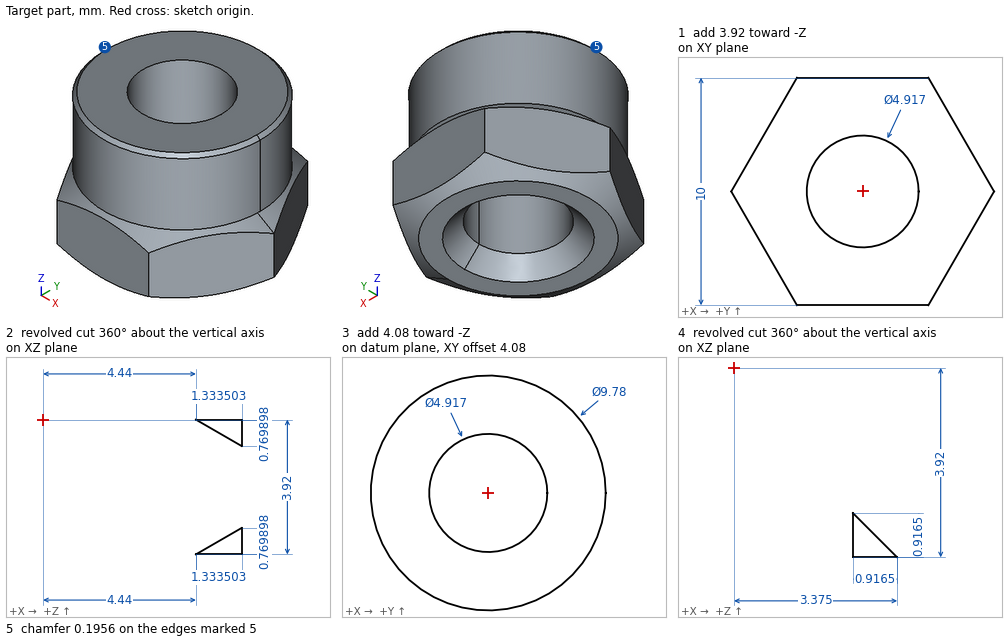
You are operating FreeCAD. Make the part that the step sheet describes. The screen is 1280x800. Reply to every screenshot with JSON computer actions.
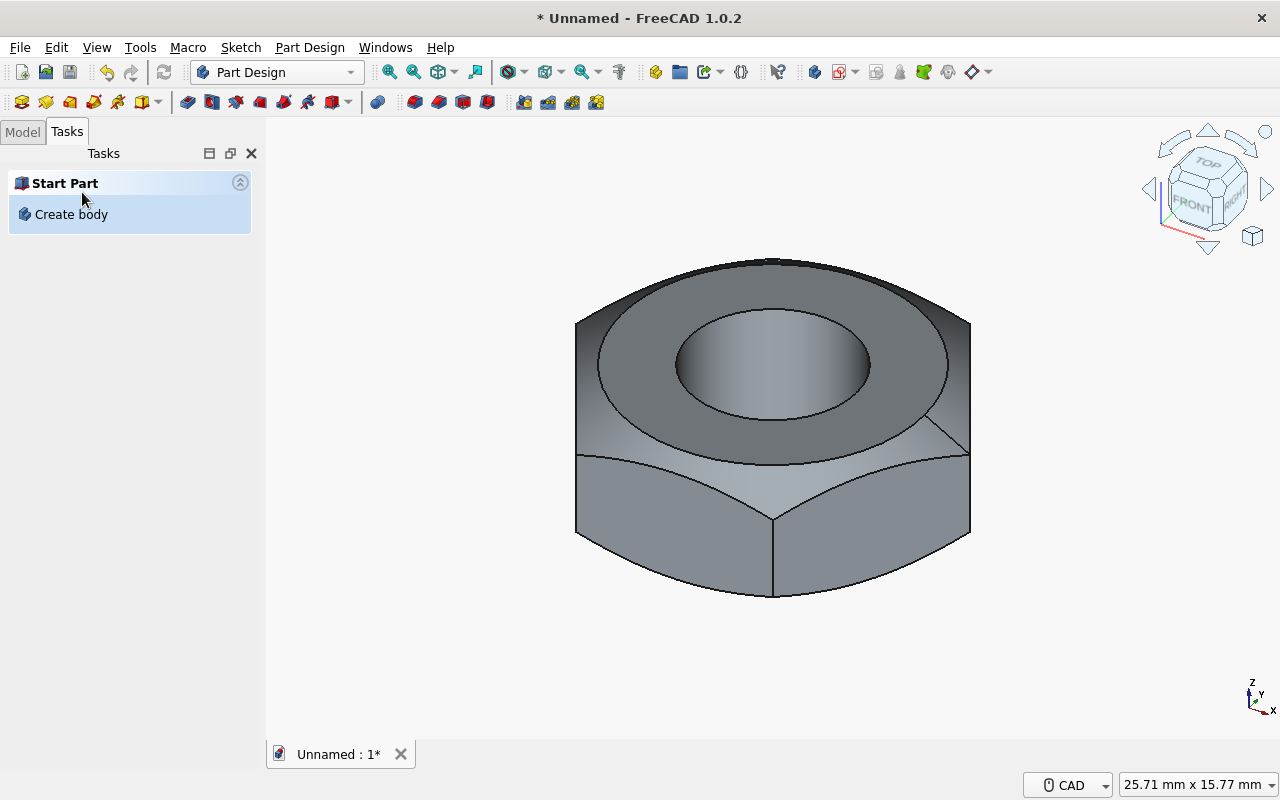
{"action": "left_click", "coordinate": [23, 131]}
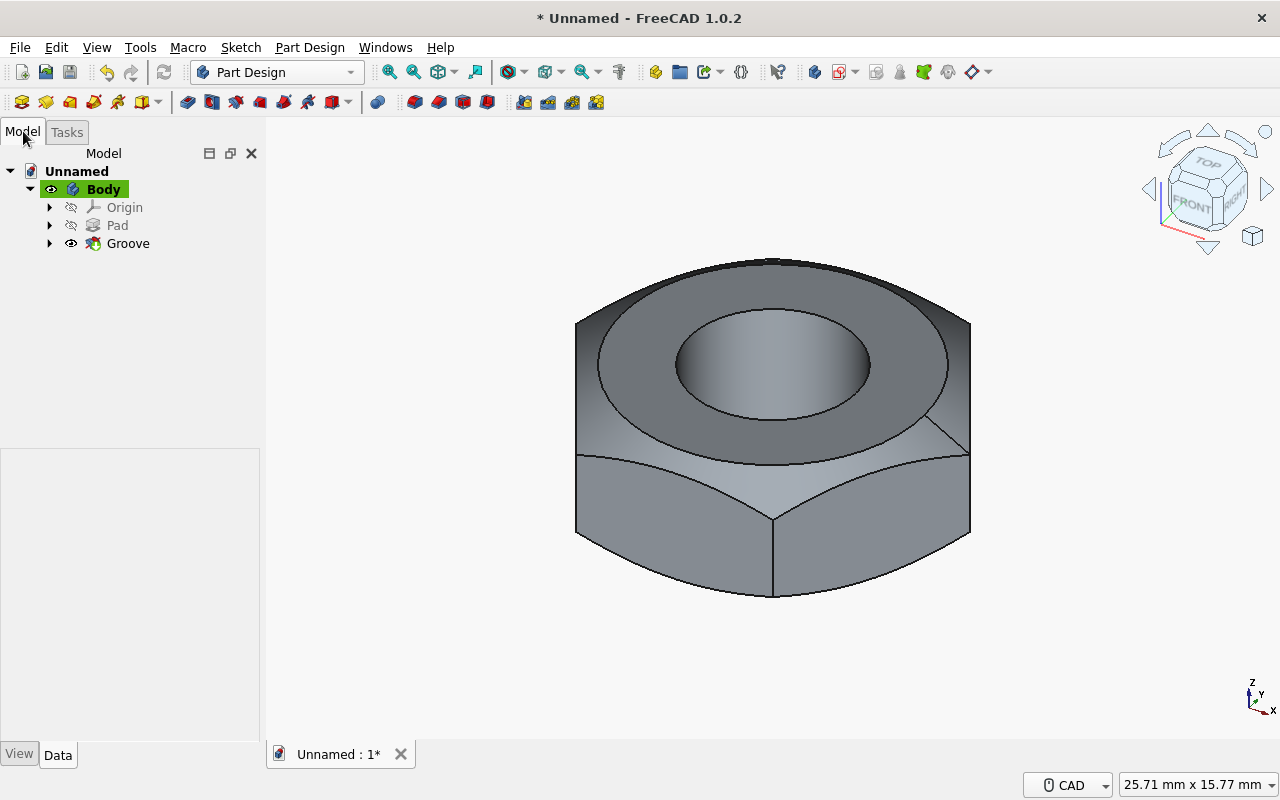
{"action": "left_click", "coordinate": [50, 207]}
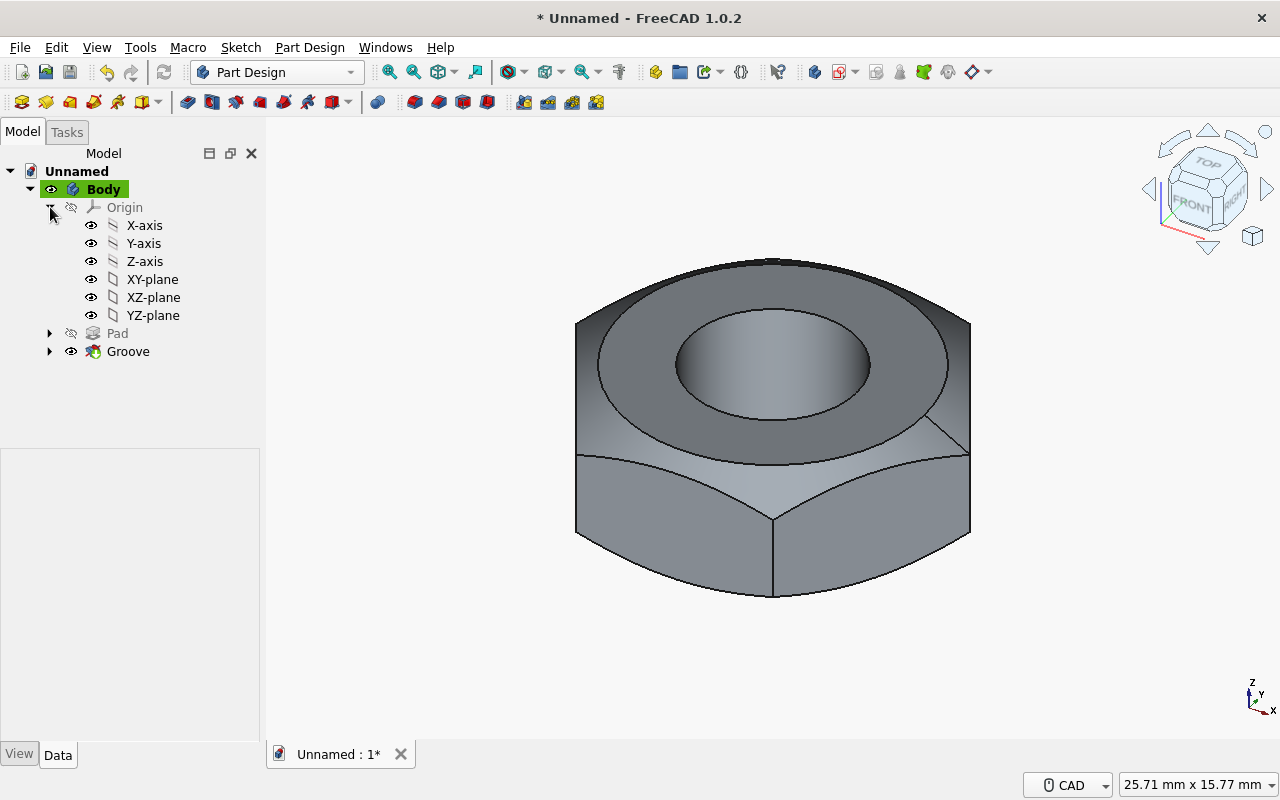
{"action": "left_click", "coordinate": [136, 279]}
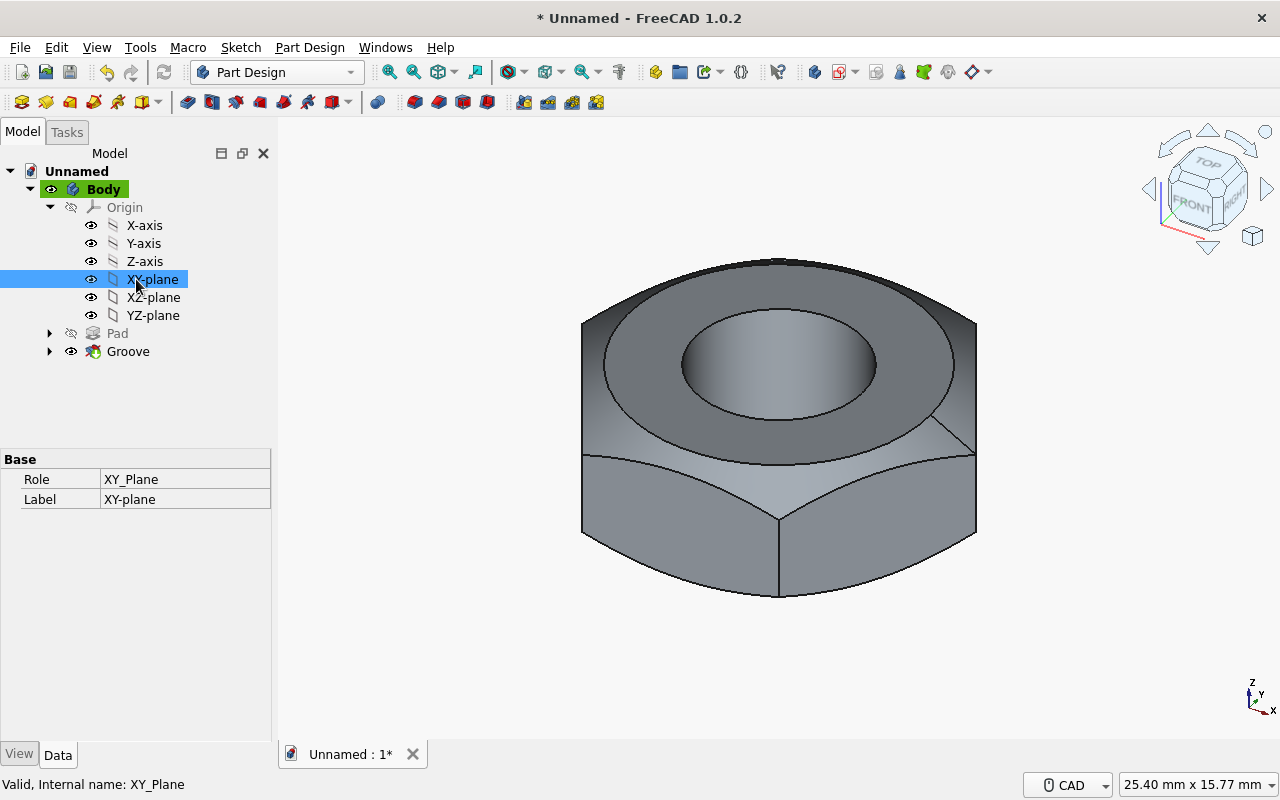
{"action": "left_click", "coordinate": [972, 72]}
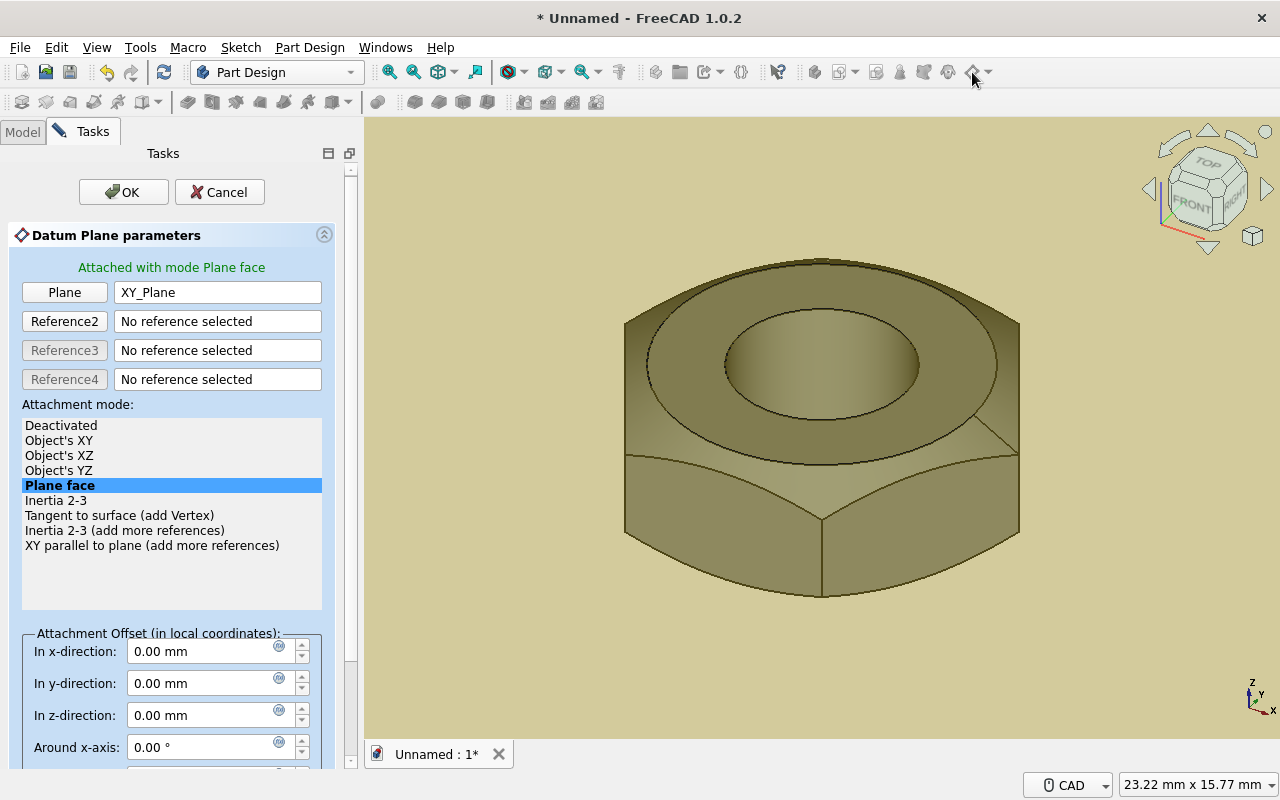
{"action": "triple_click", "coordinate": [210, 715]}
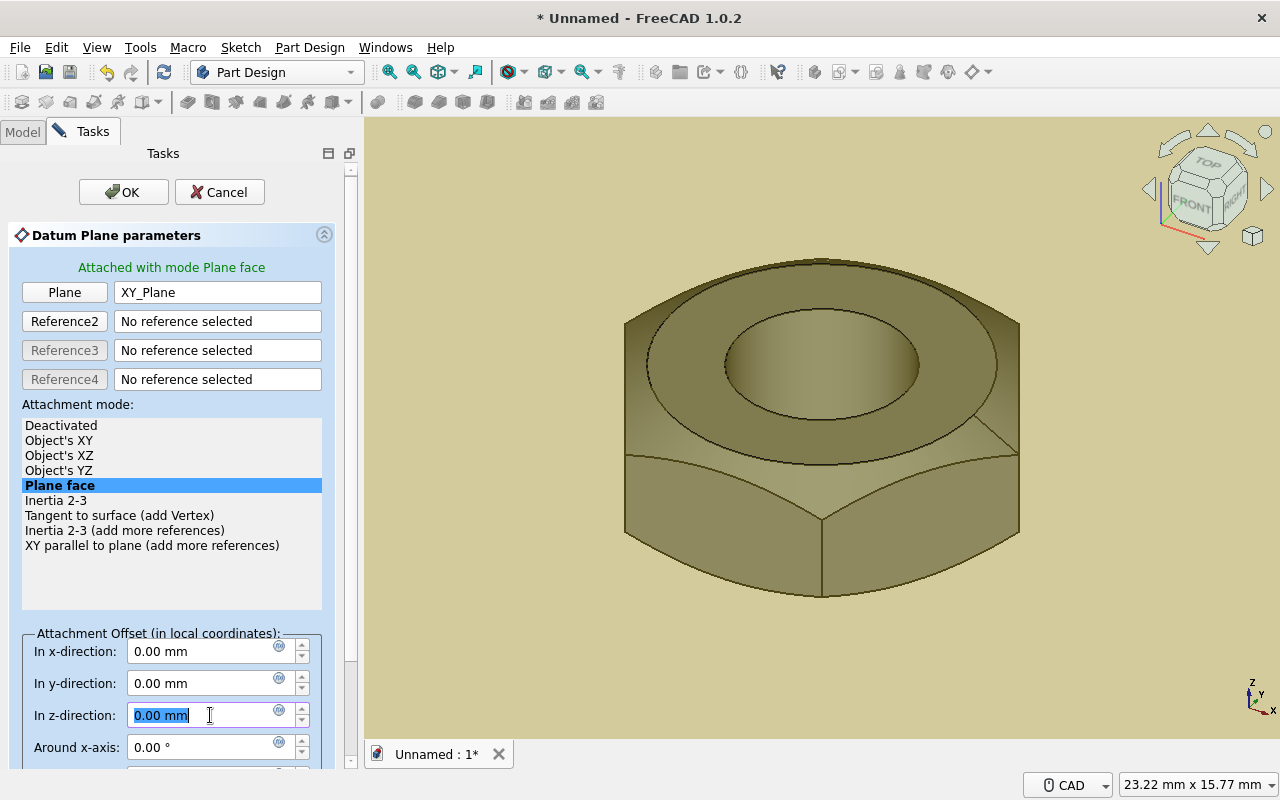
{"action": "type", "text": "4.08"}
{"action": "key", "text": "Tab"}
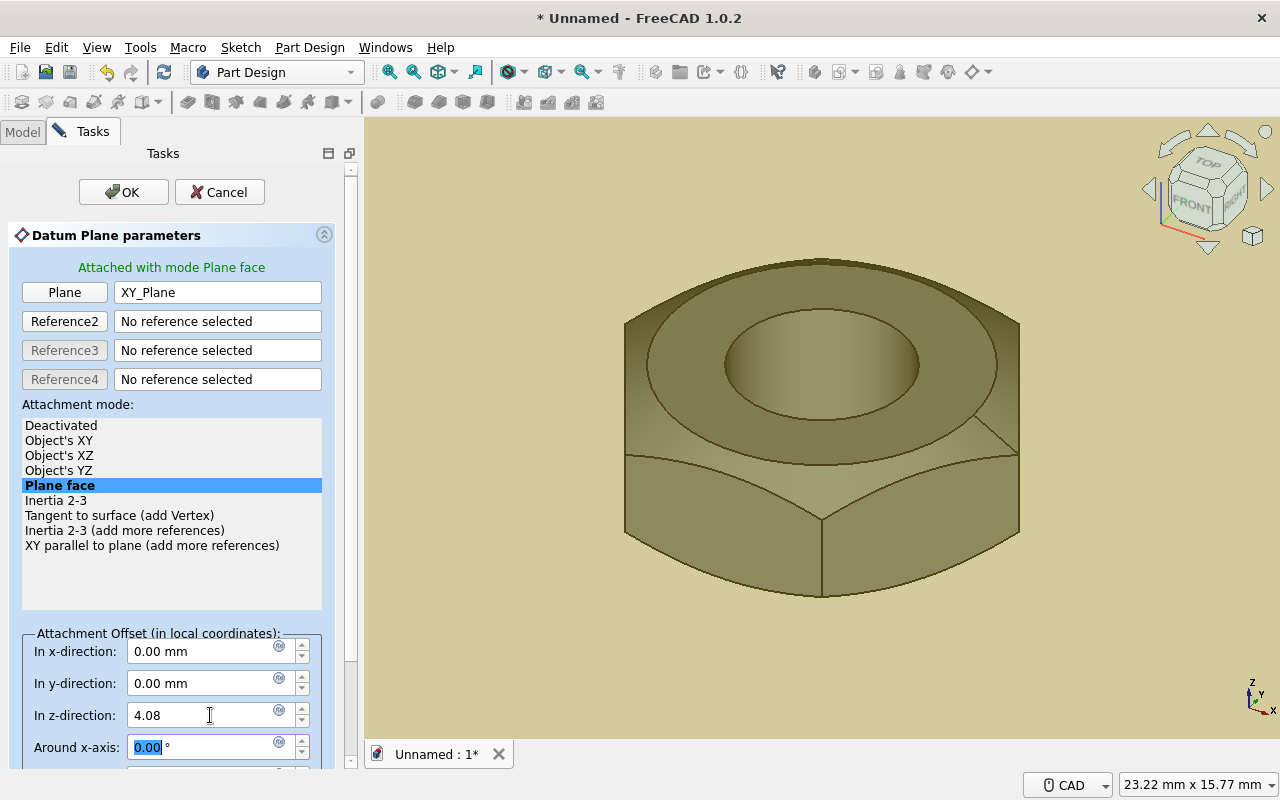
{"action": "left_click", "coordinate": [124, 192]}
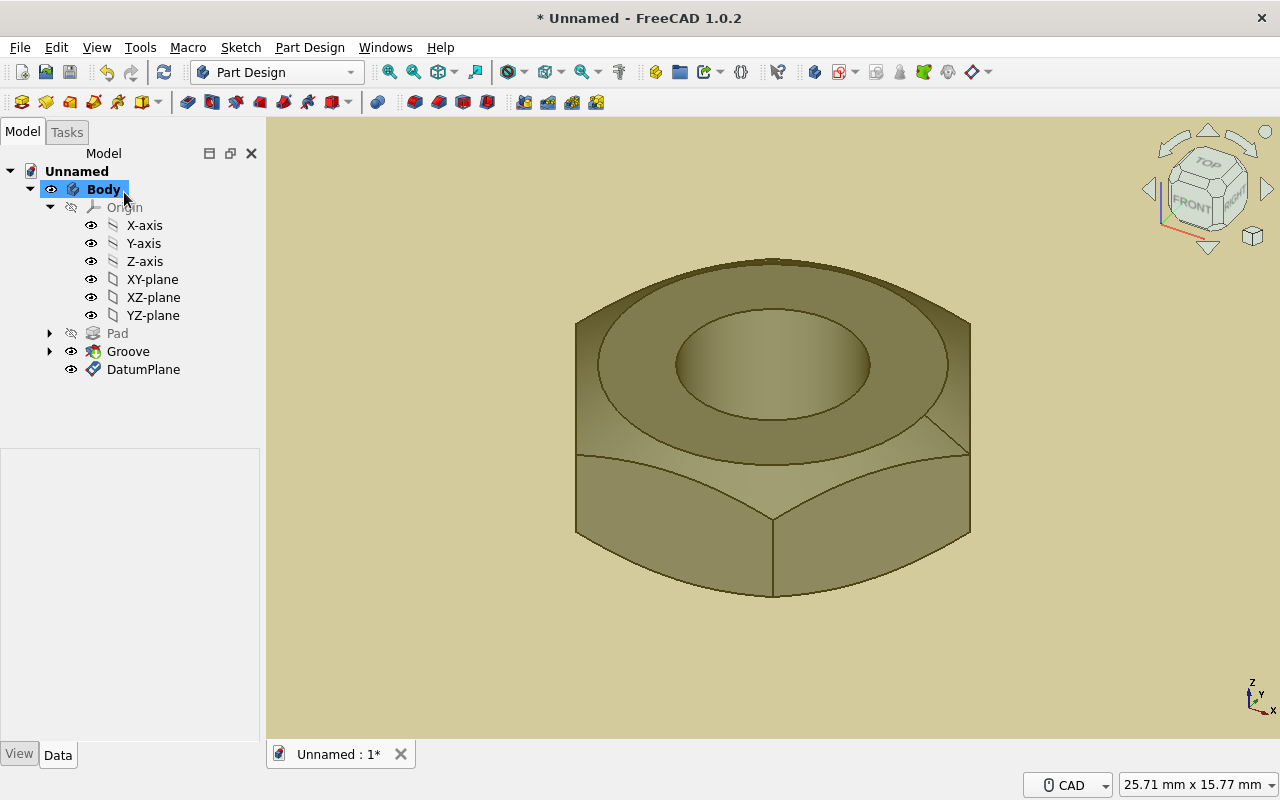
{"action": "left_click", "coordinate": [116, 369]}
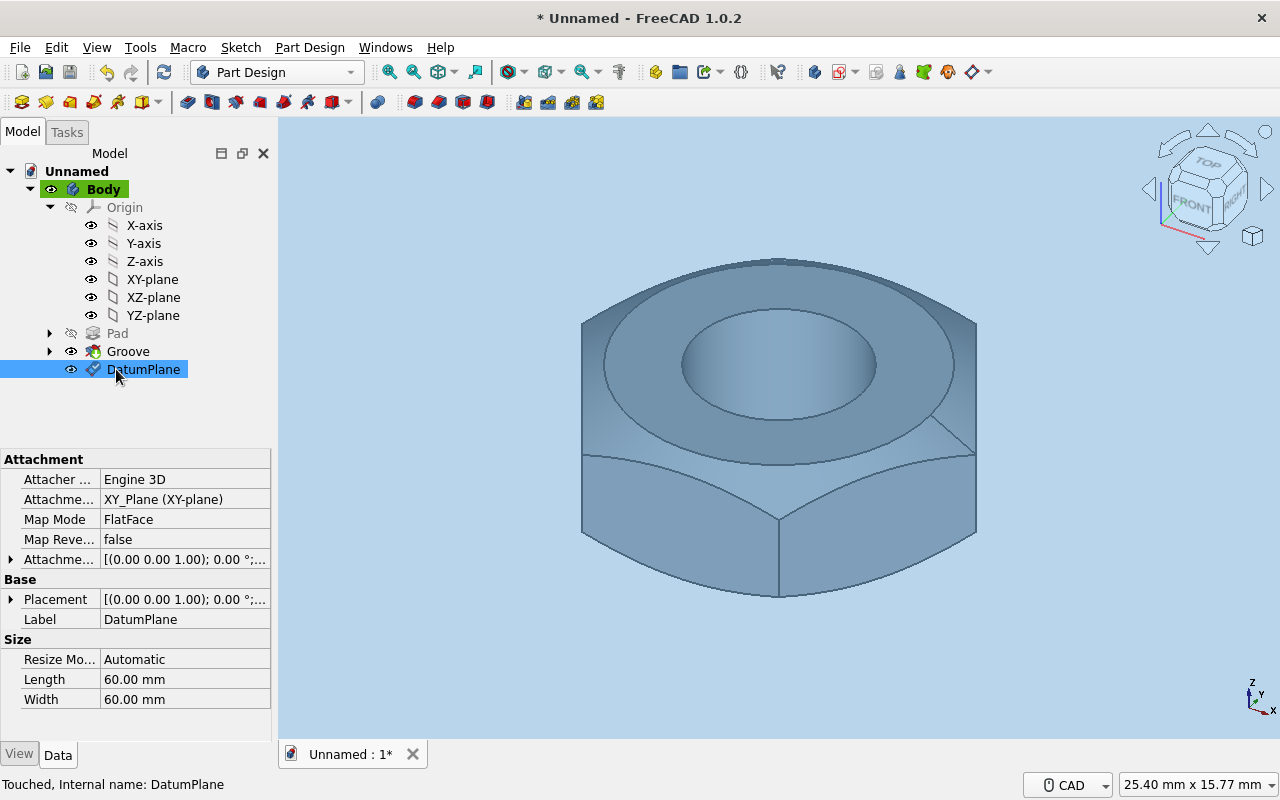
{"action": "left_click", "coordinate": [840, 72]}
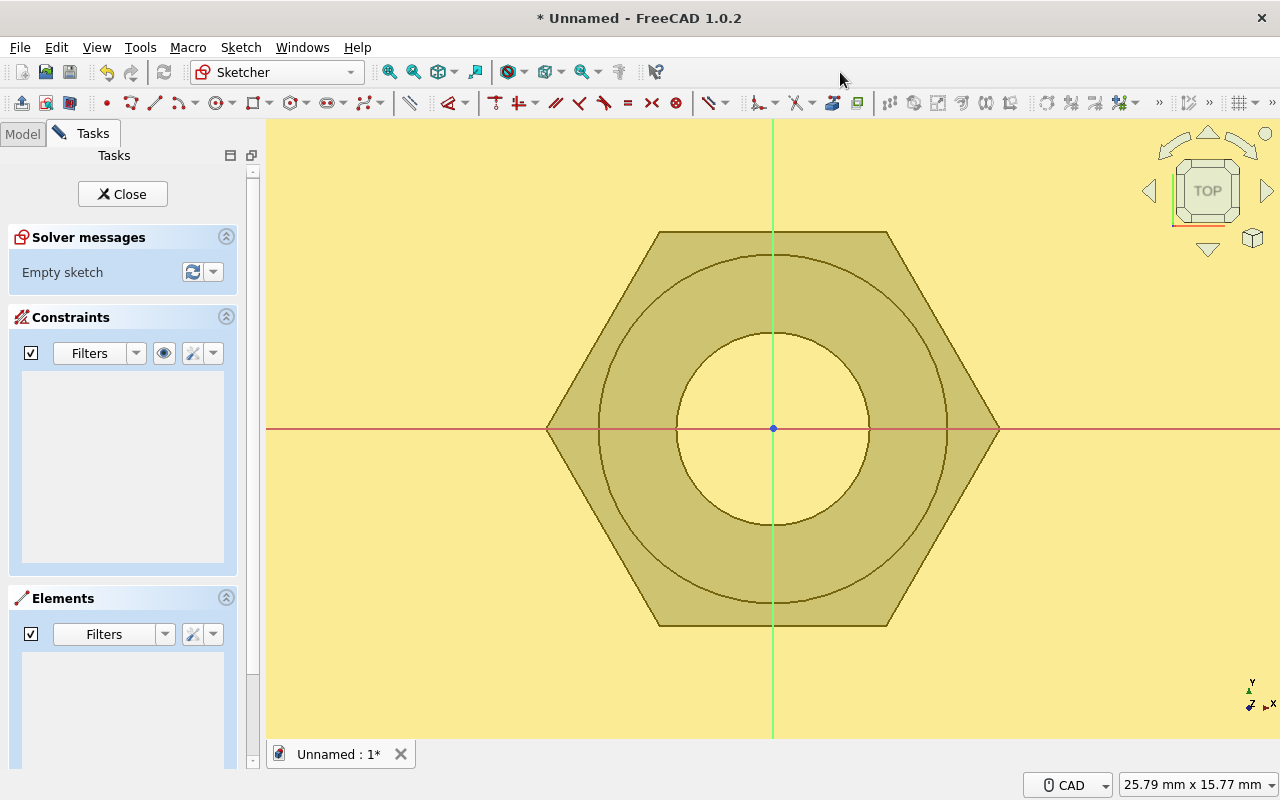
{"action": "key", "text": "g c"}